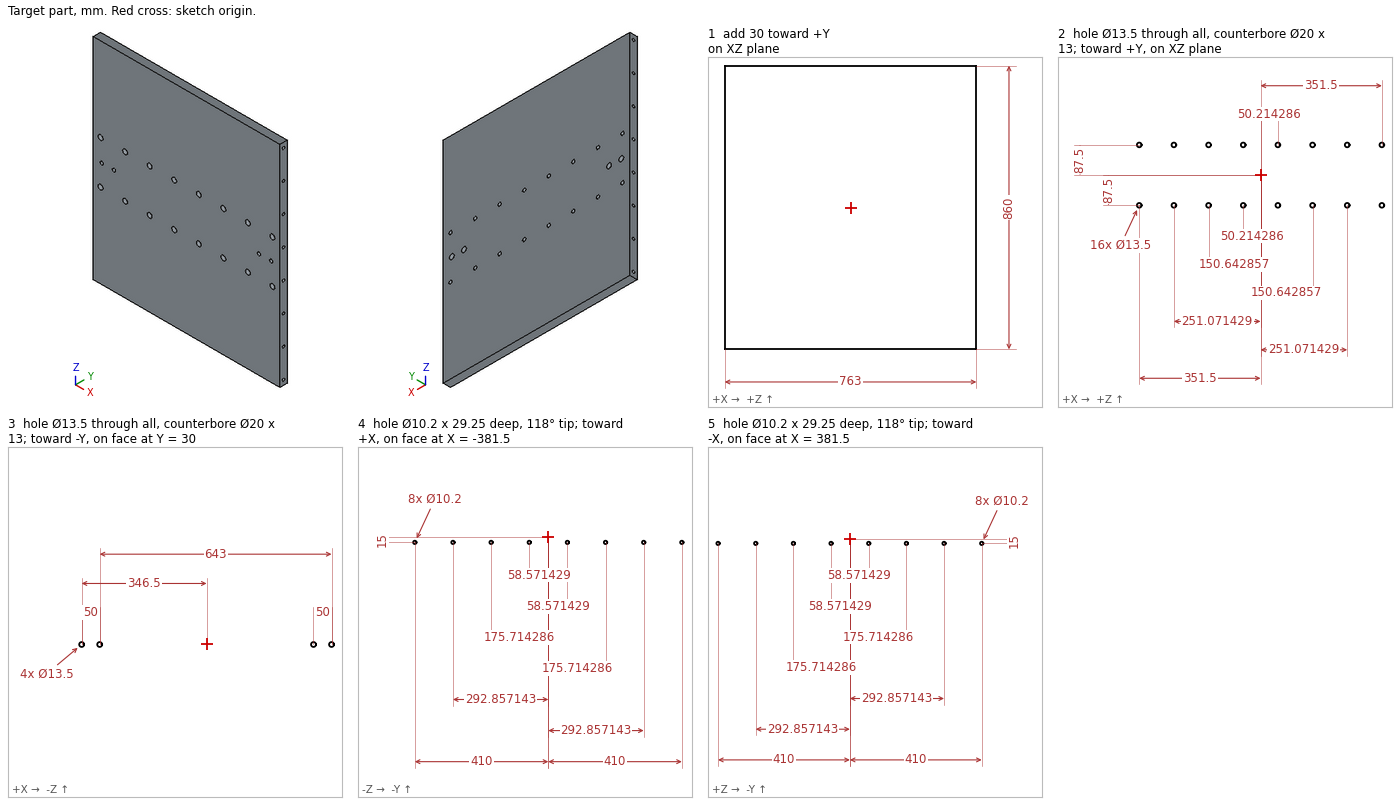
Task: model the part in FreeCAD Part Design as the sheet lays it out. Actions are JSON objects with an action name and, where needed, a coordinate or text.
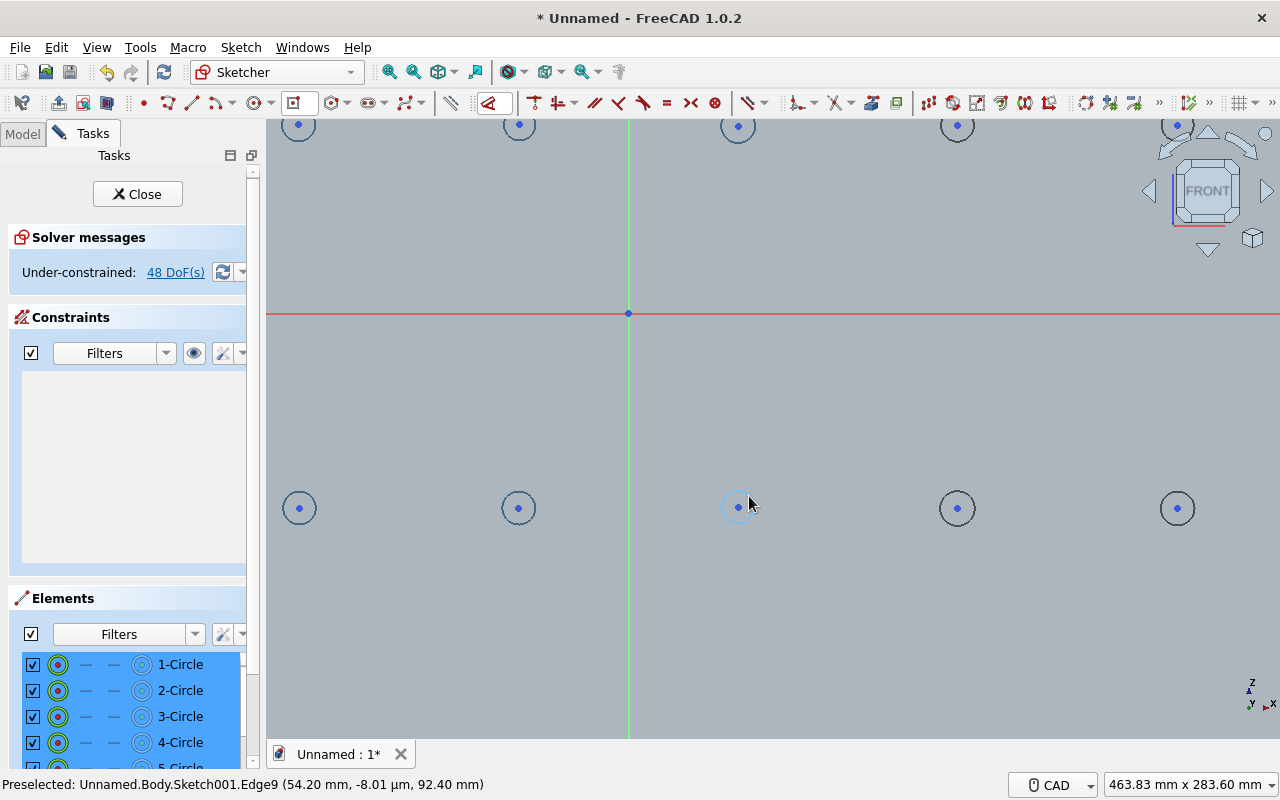
{"action": "left_click", "coordinate": [749, 496]}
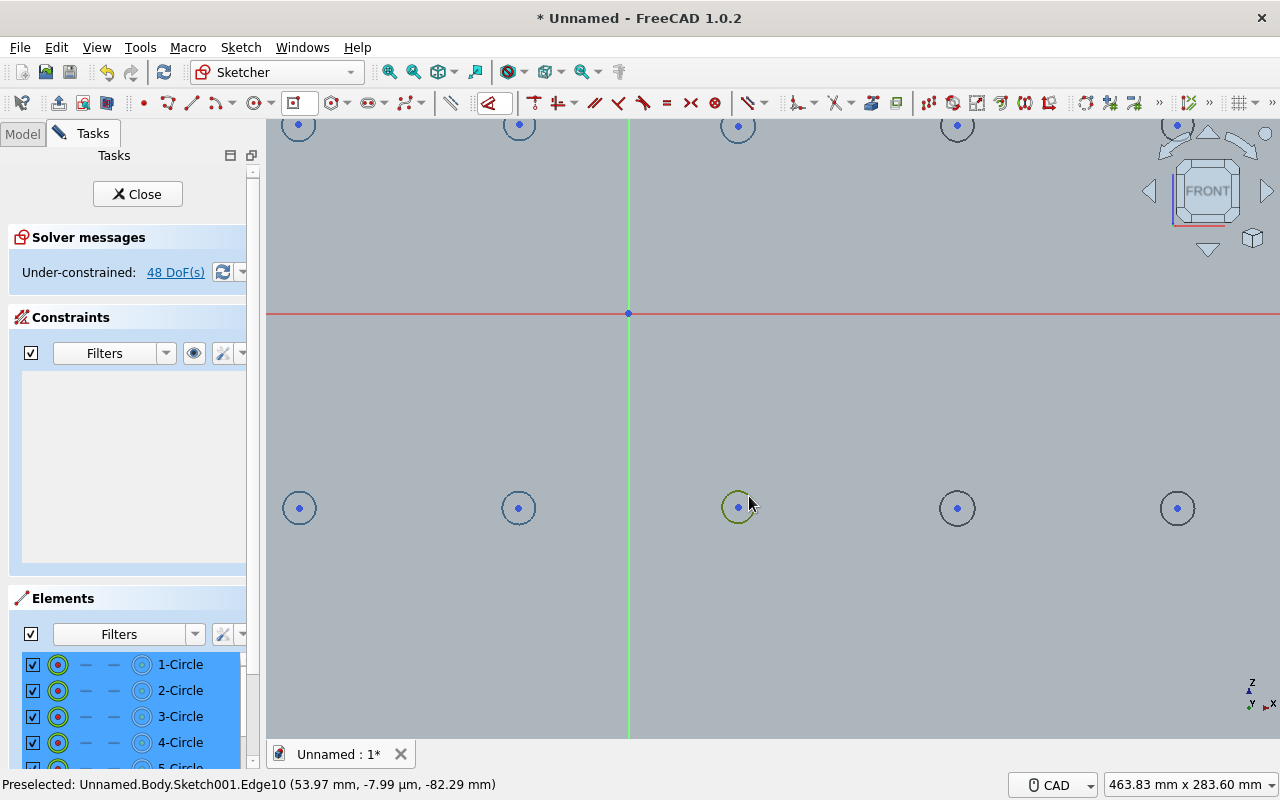
{"action": "left_click", "coordinate": [970, 496]}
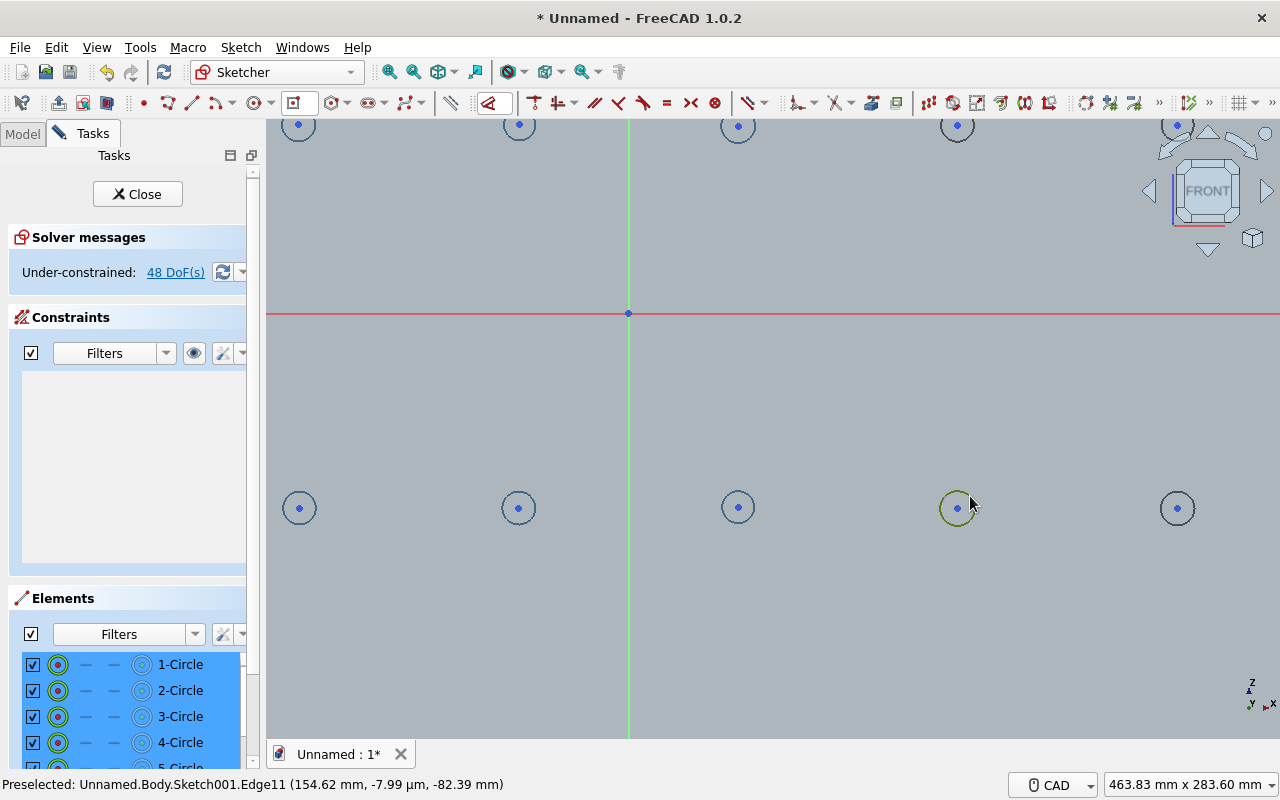
{"action": "scroll", "coordinate": [749, 496], "scroll_direction": "down", "scroll_amount": 5}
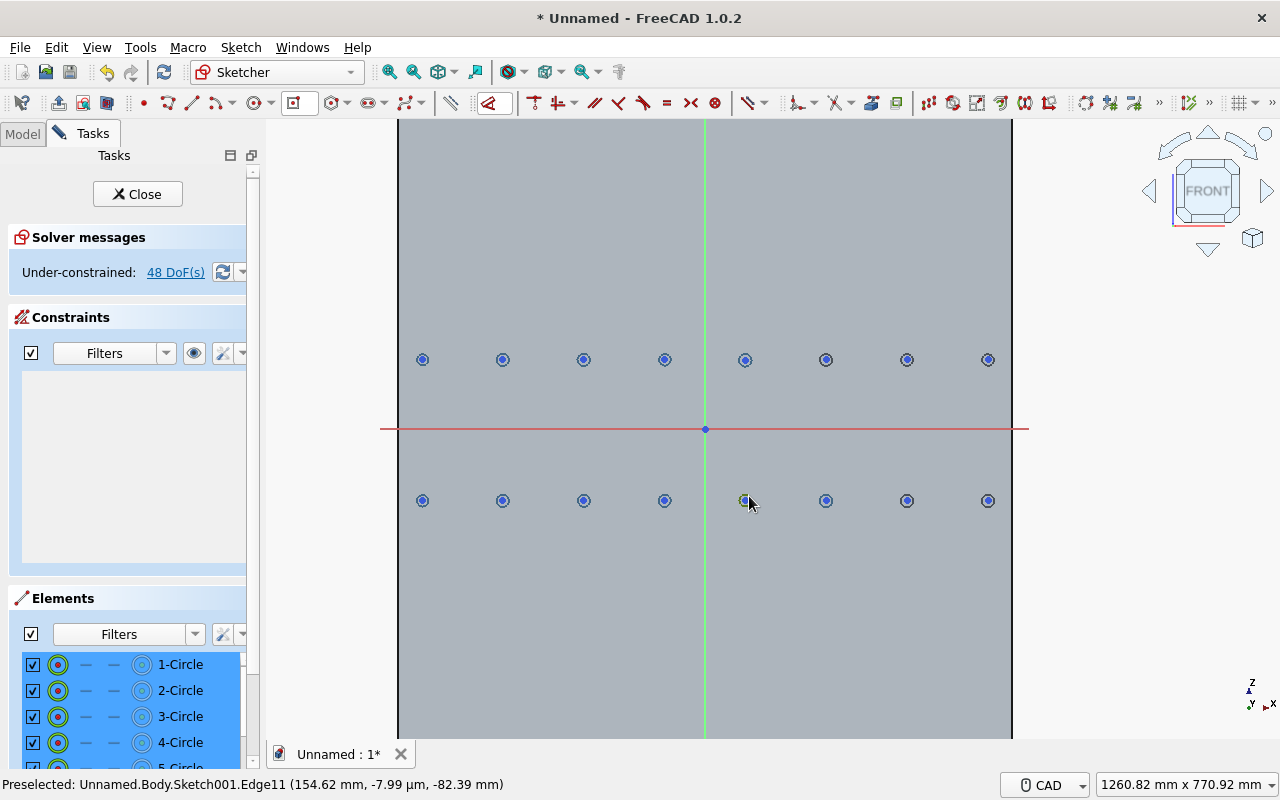
{"action": "scroll", "coordinate": [830, 356], "scroll_direction": "up", "scroll_amount": 5}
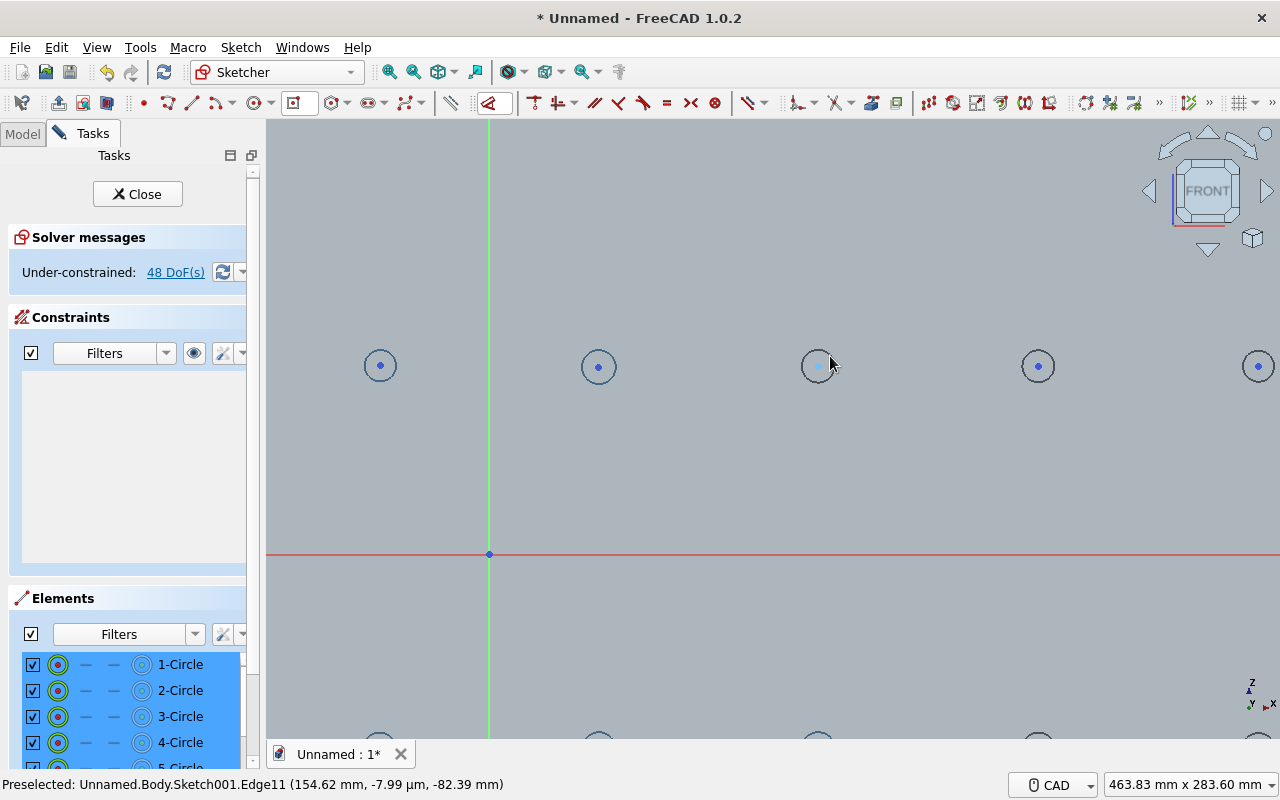
{"action": "left_click", "coordinate": [830, 355]}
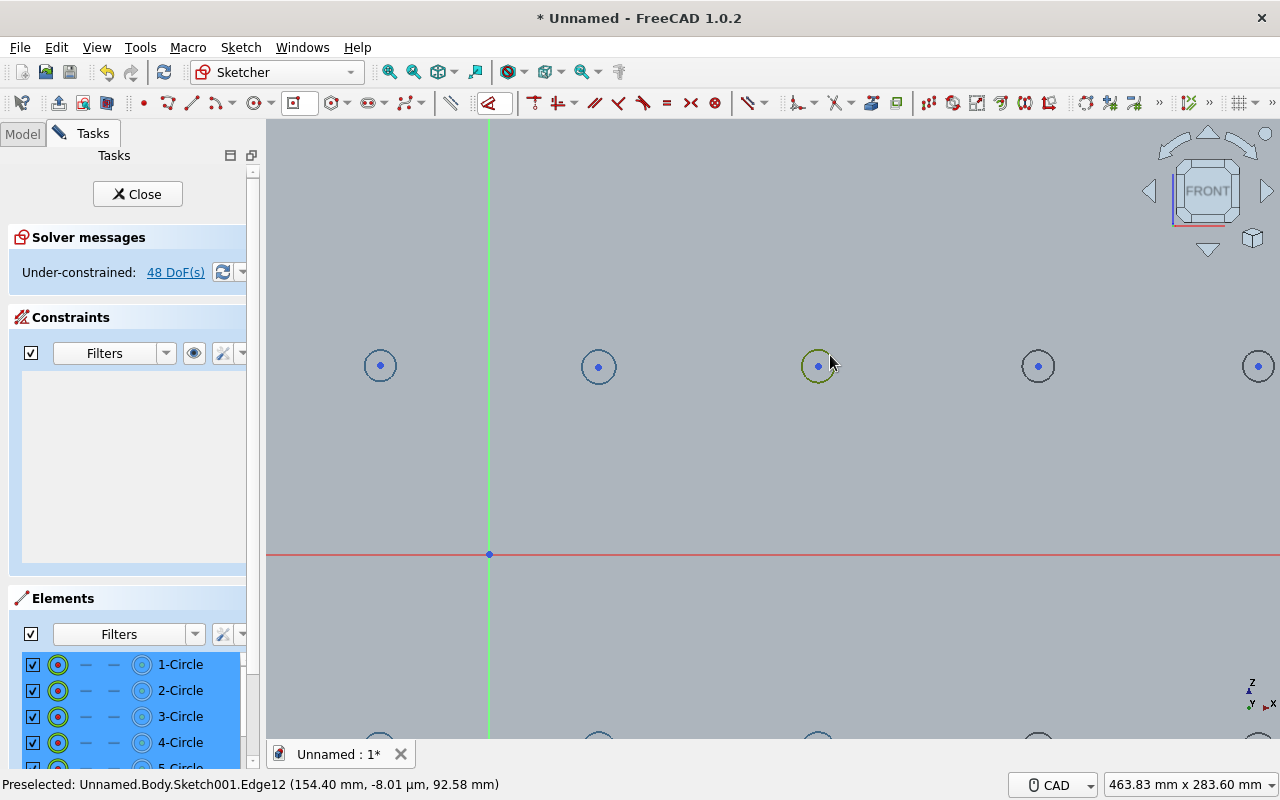
{"action": "scroll", "coordinate": [830, 356], "scroll_direction": "down", "scroll_amount": 5}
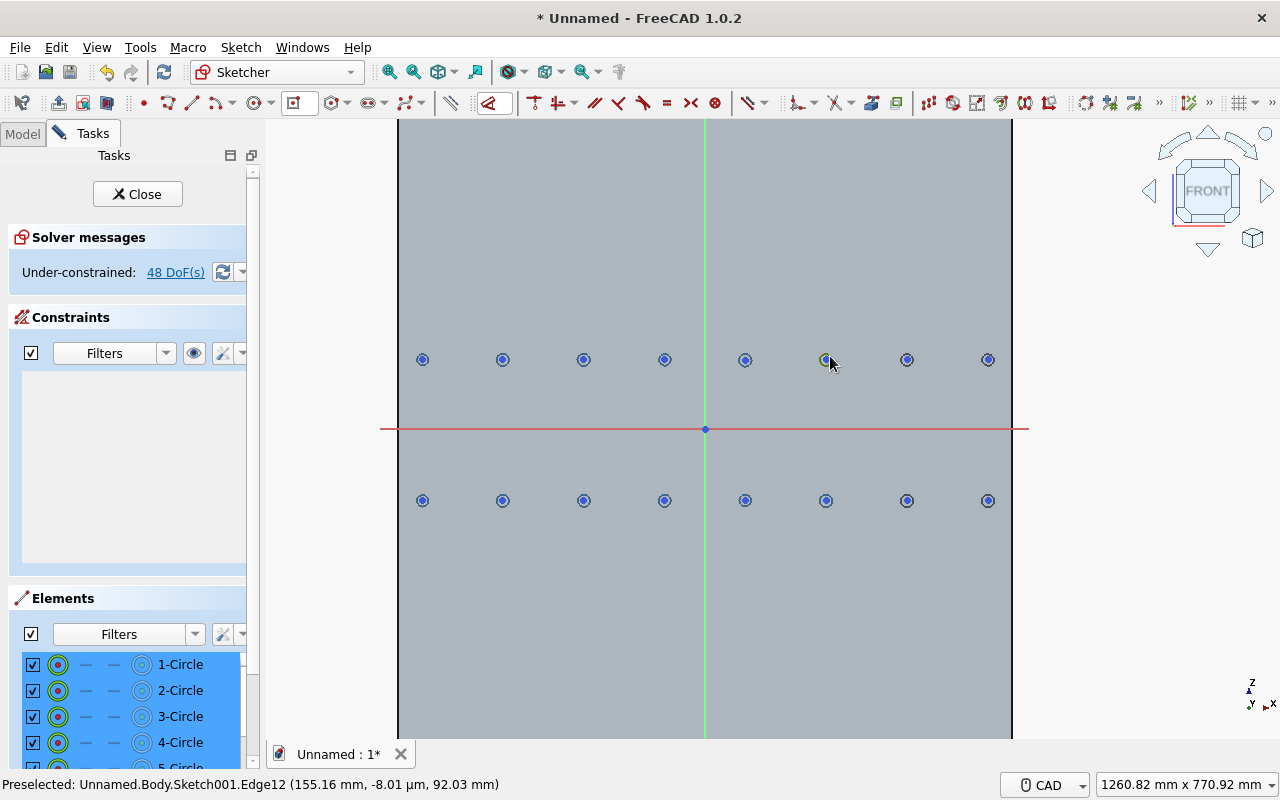
{"action": "scroll", "coordinate": [911, 497], "scroll_direction": "up", "scroll_amount": 4}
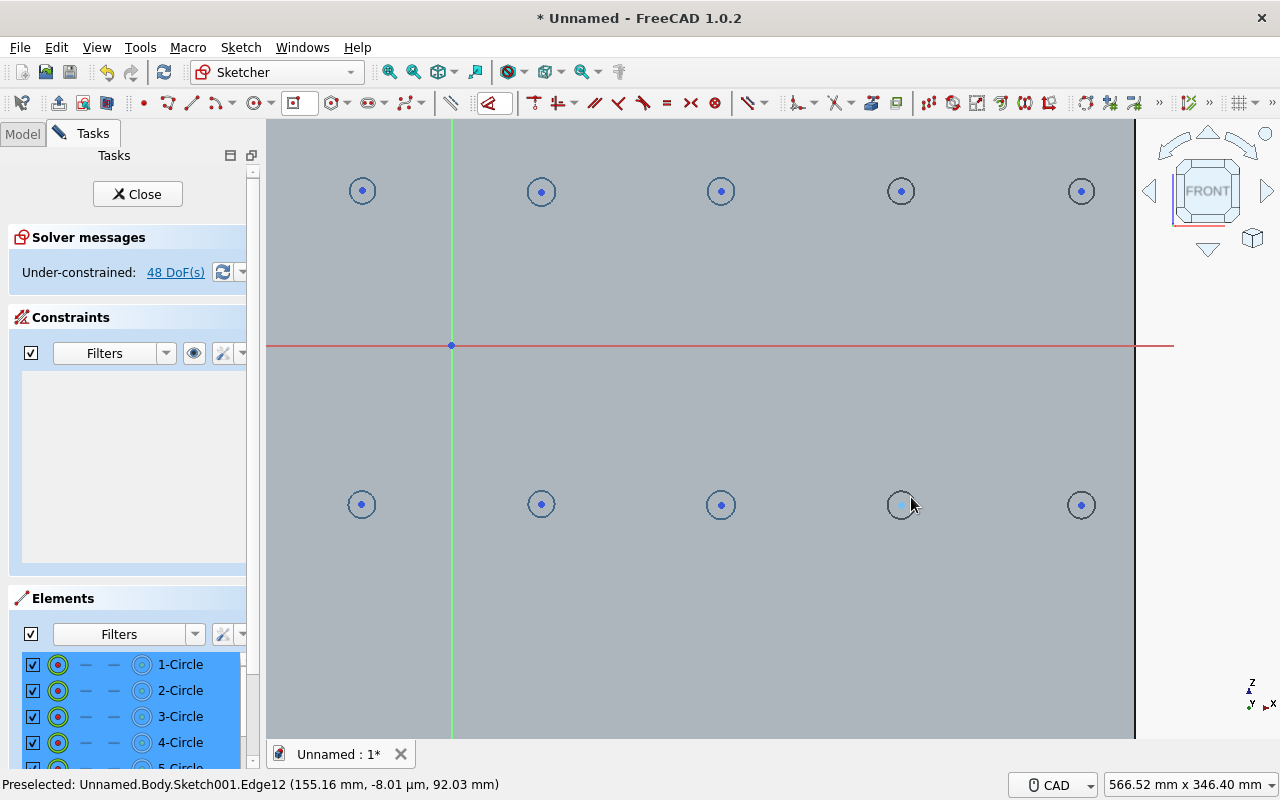
{"action": "left_click", "coordinate": [911, 495]}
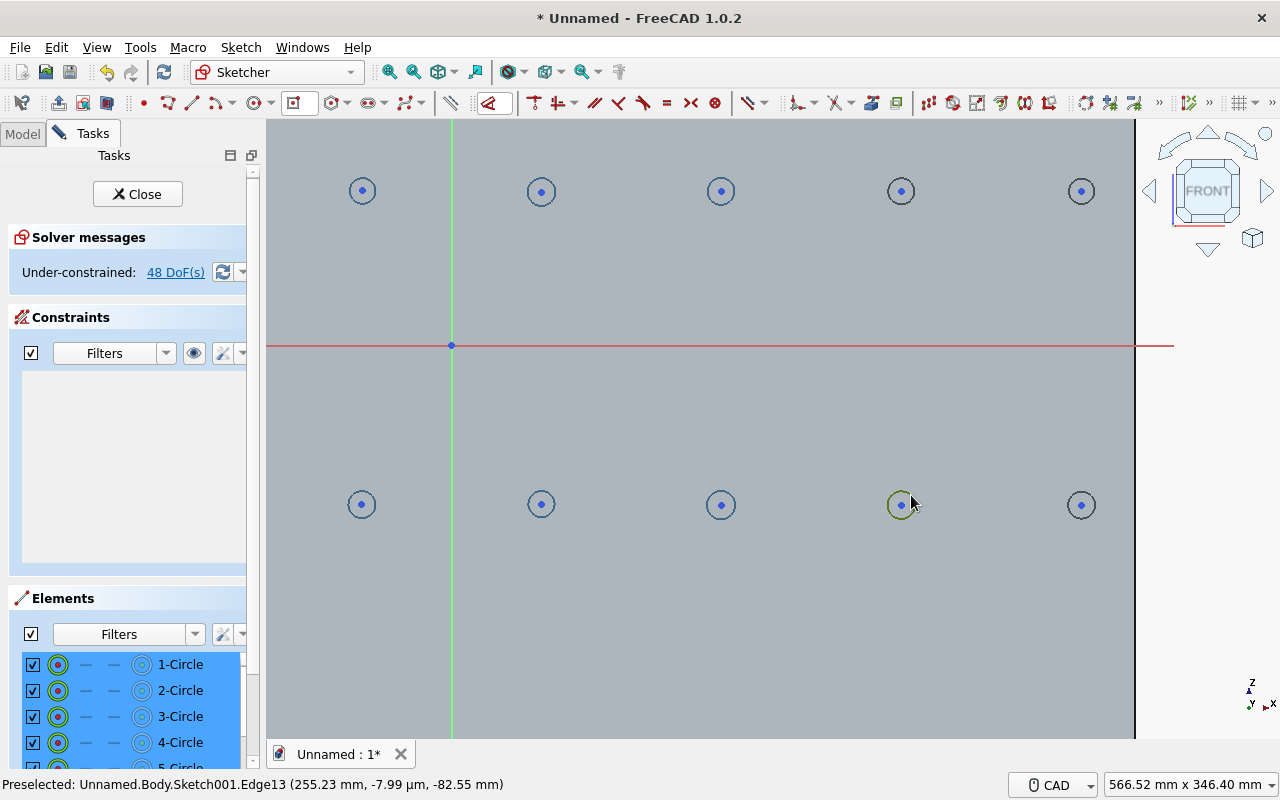
{"action": "left_click", "coordinate": [911, 182]}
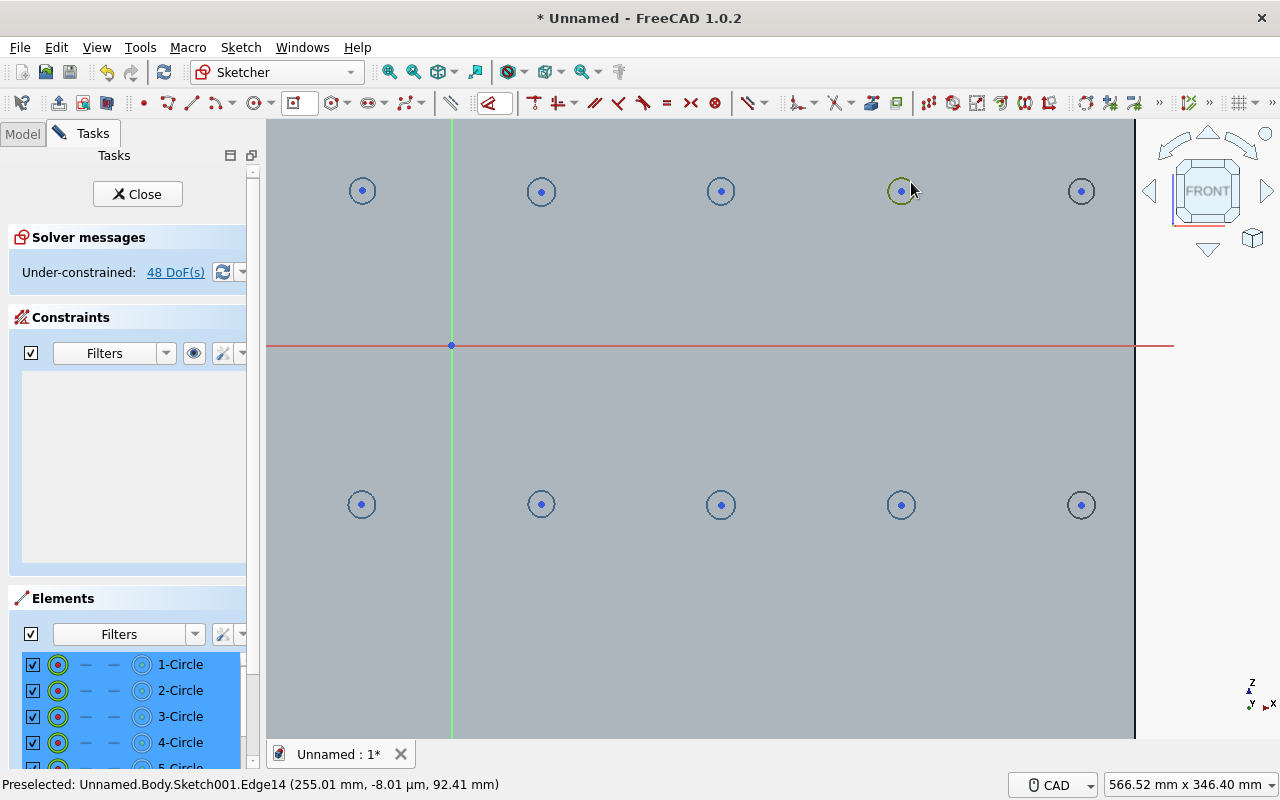
{"action": "left_click", "coordinate": [1091, 182]}